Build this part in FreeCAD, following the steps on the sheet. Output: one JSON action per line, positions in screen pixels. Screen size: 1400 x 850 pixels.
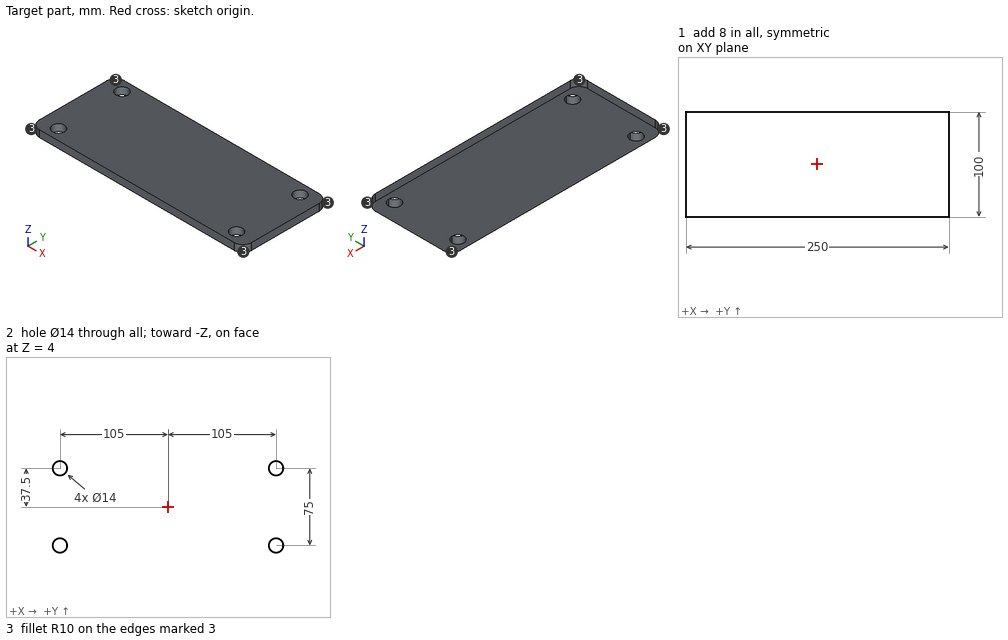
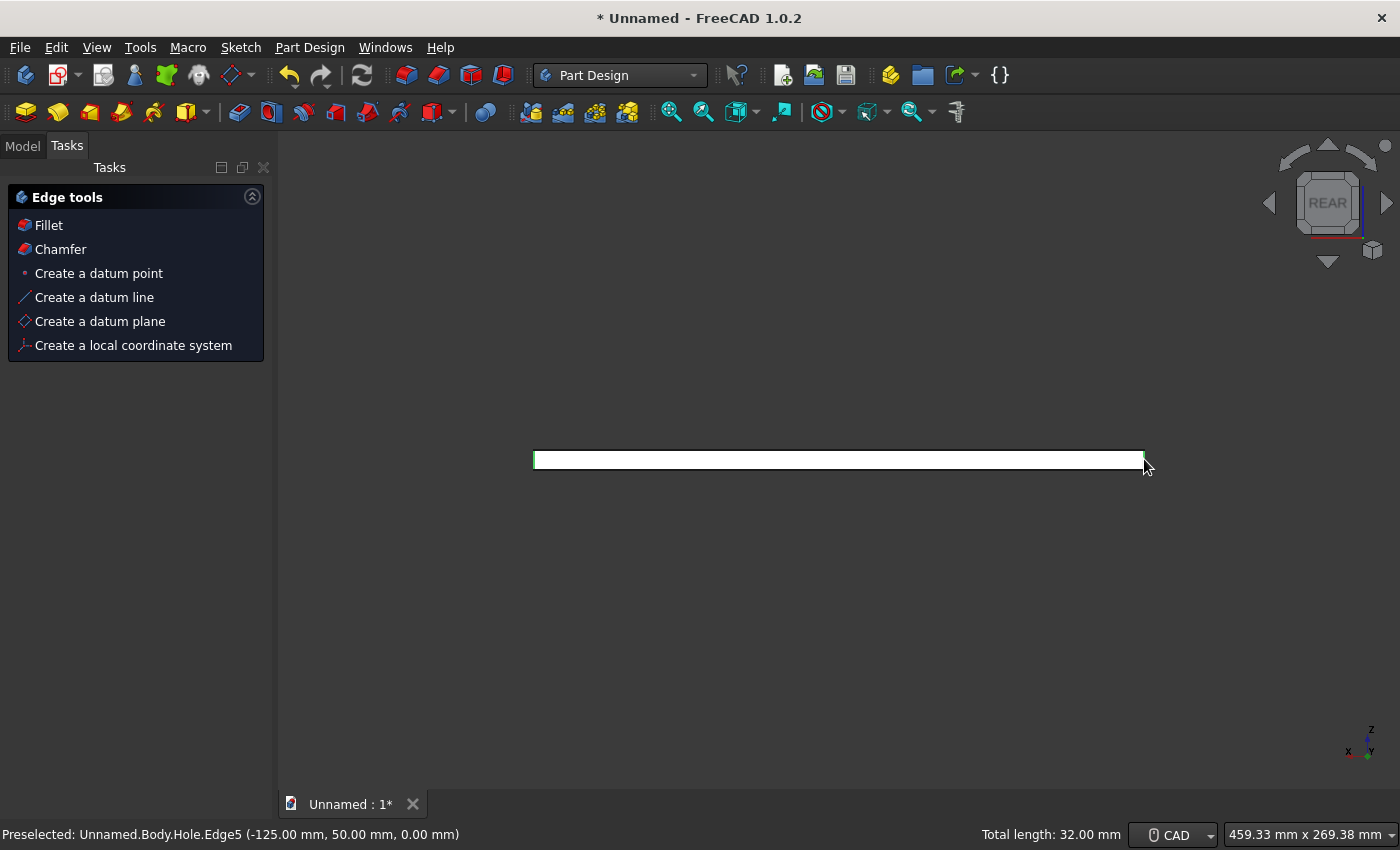
{"action": "left_click", "coordinate": [408, 76]}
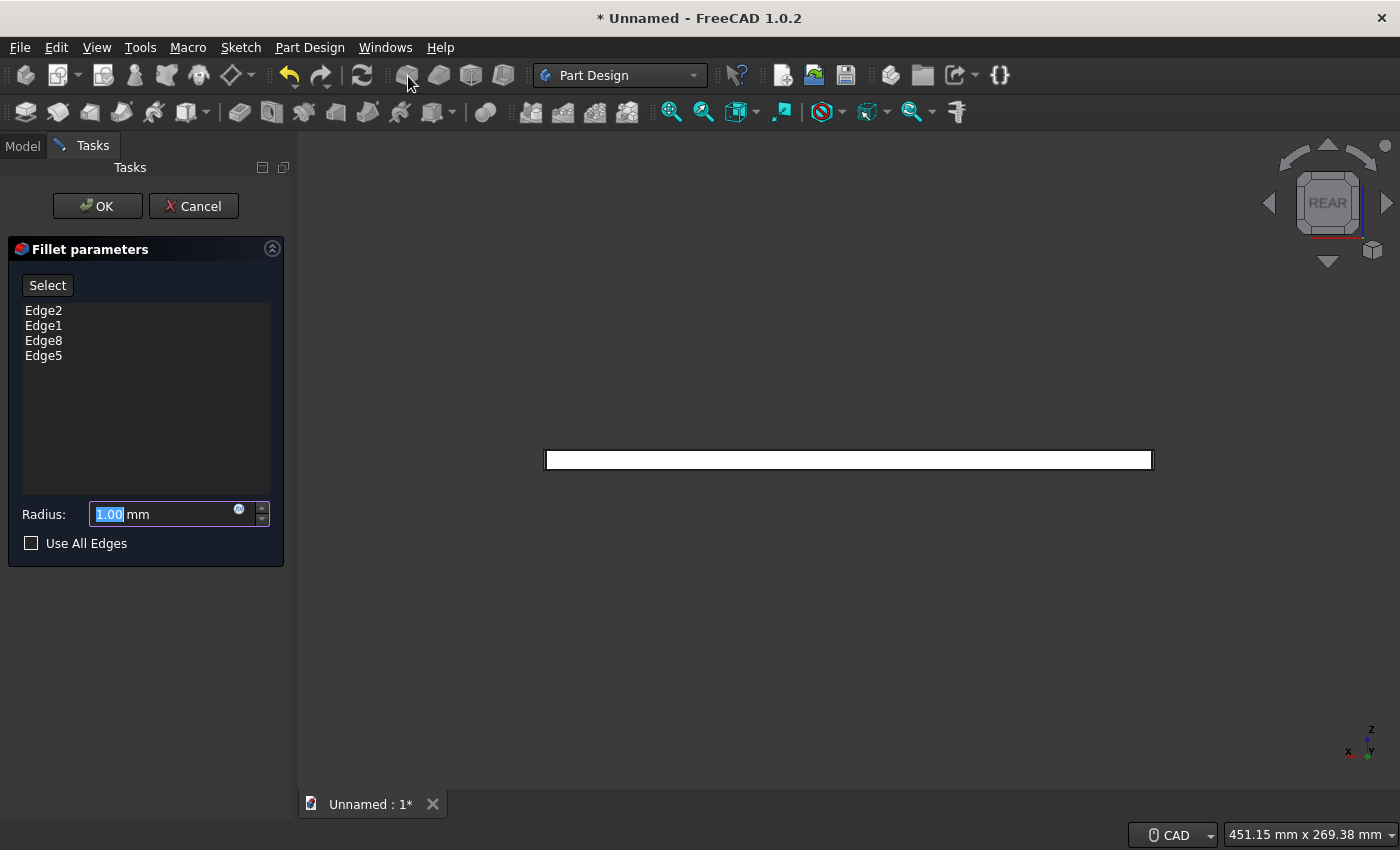
{"action": "type", "text": "10"}
{"action": "key", "text": "Tab"}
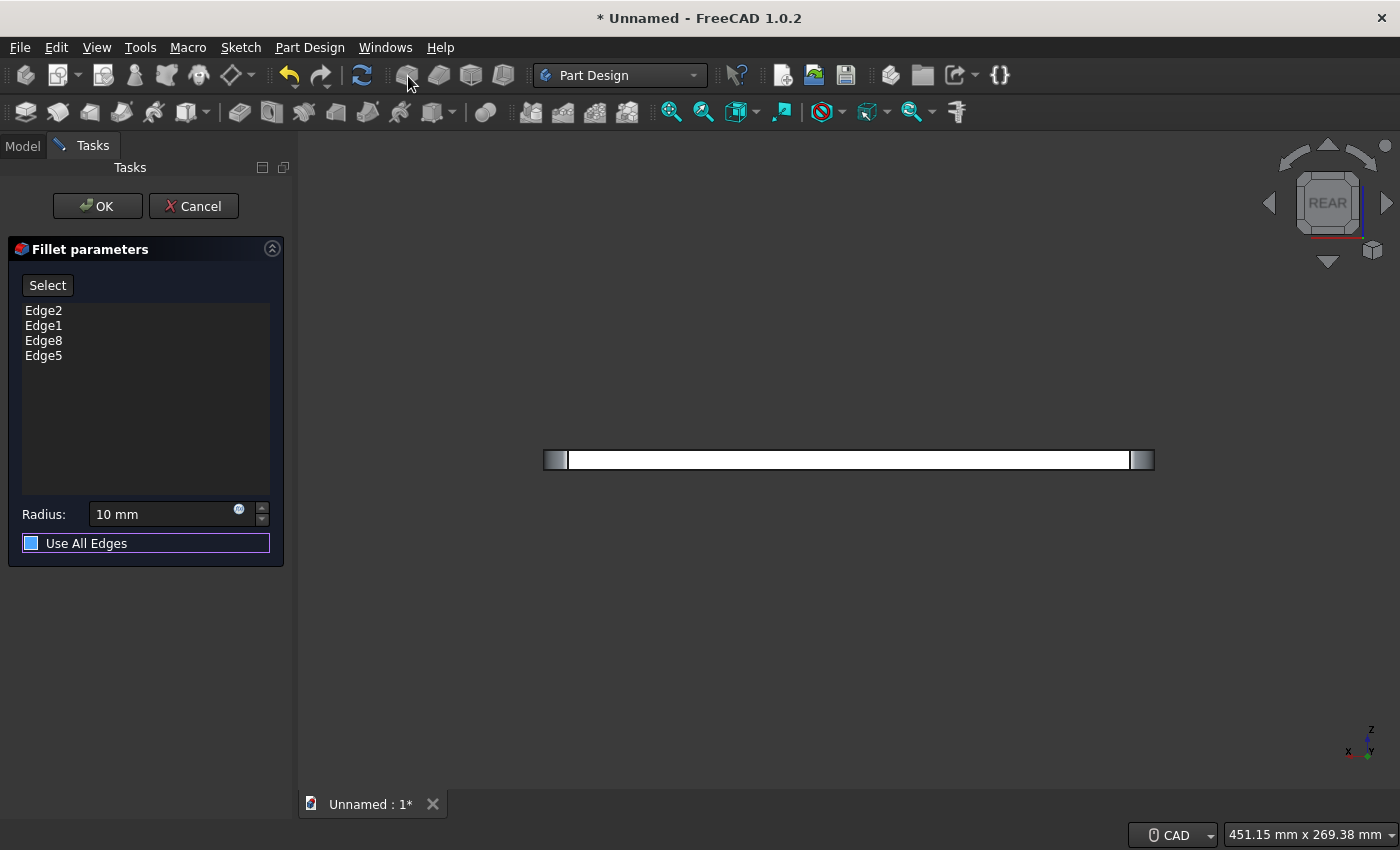
{"action": "left_click", "coordinate": [98, 206]}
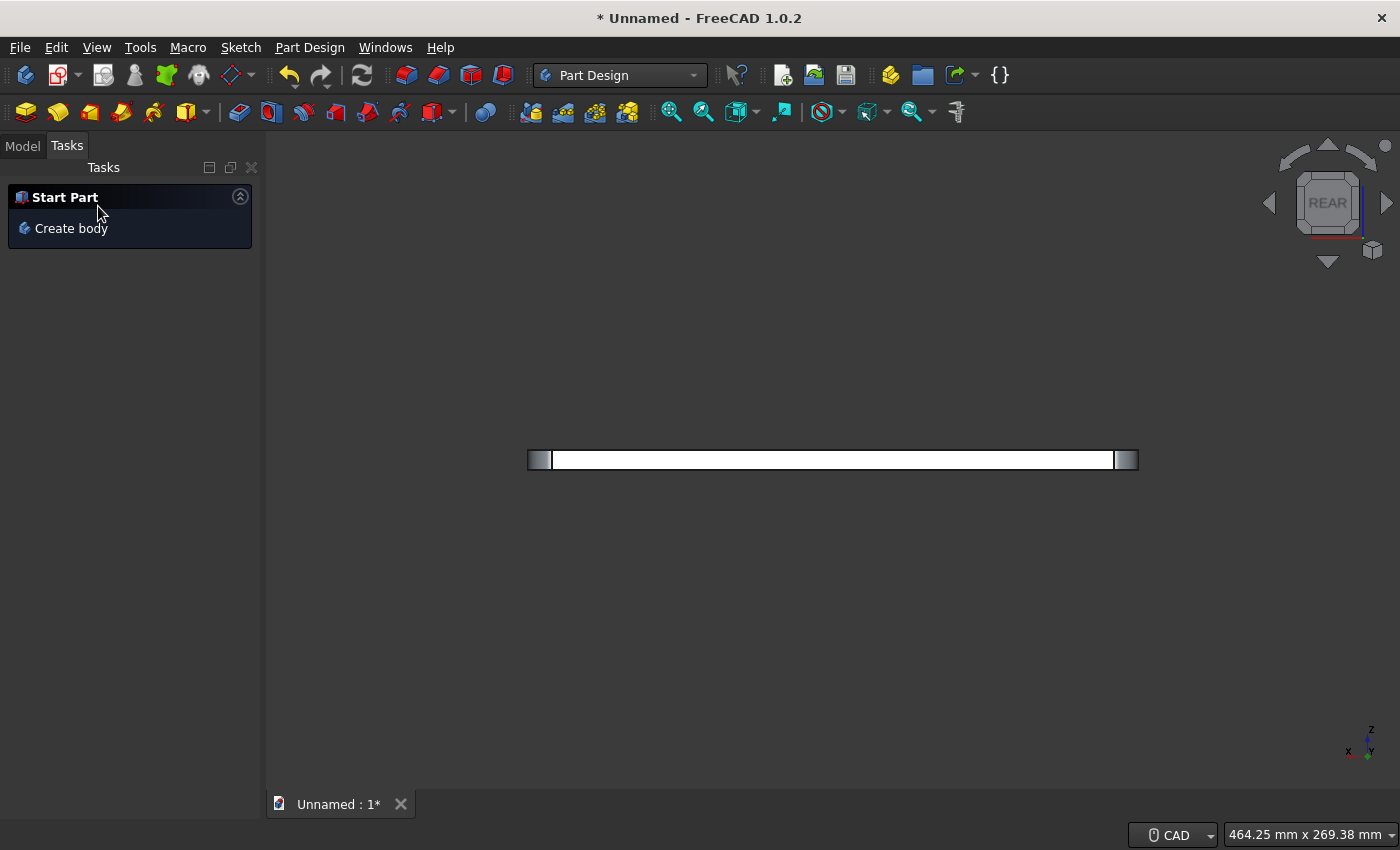
{"action": "key", "text": "0"}